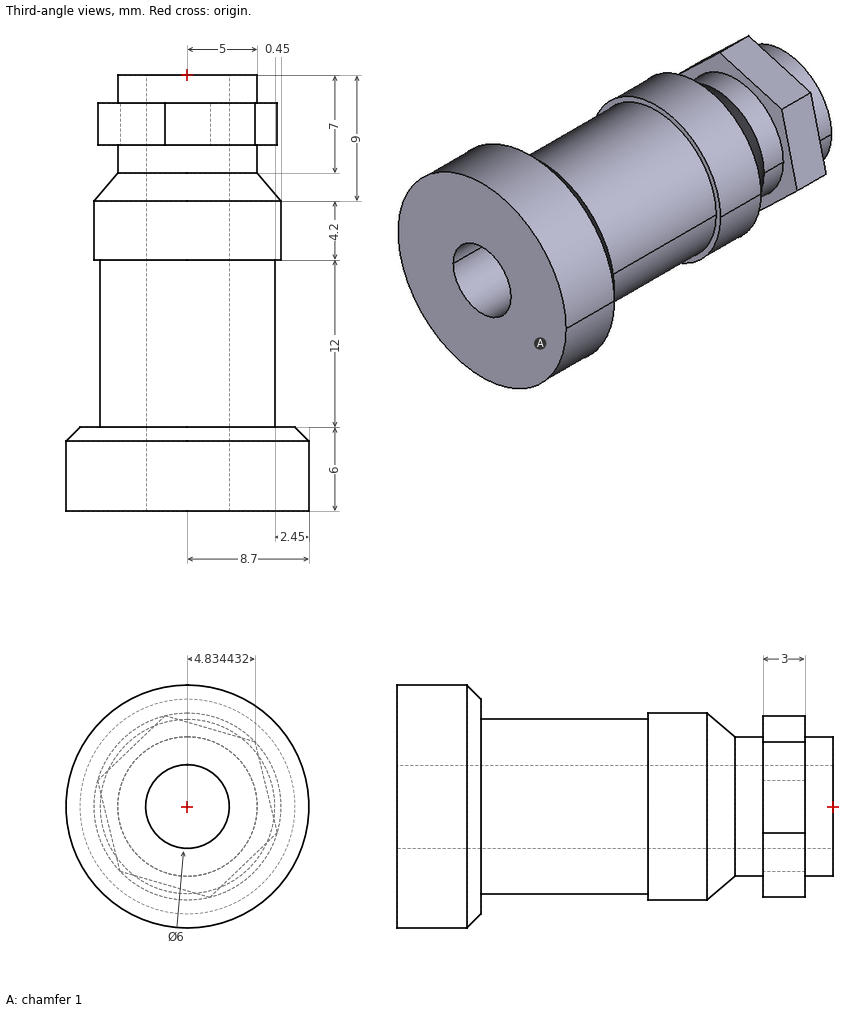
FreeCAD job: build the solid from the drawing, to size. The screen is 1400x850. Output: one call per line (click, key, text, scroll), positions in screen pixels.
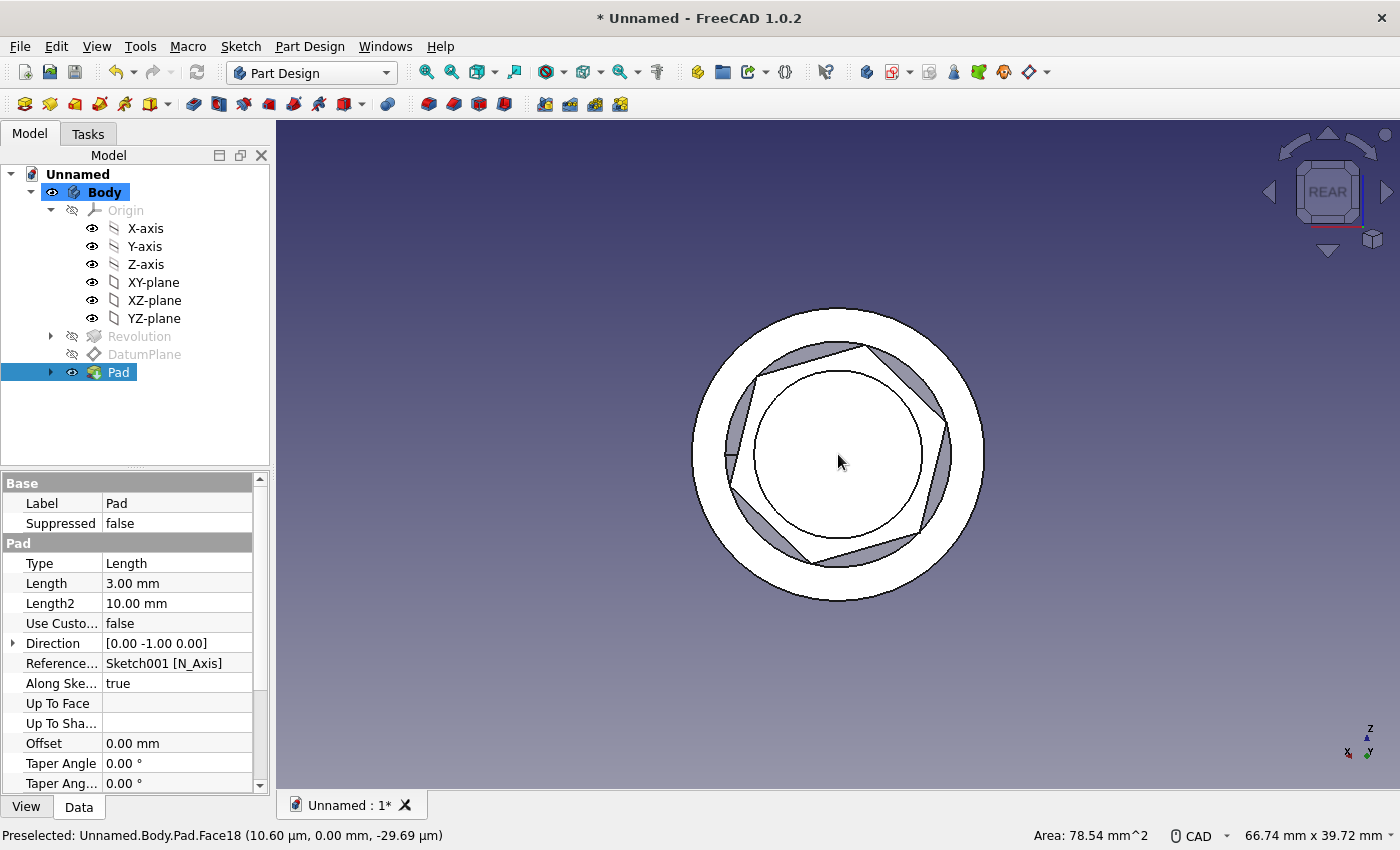
click(892, 72)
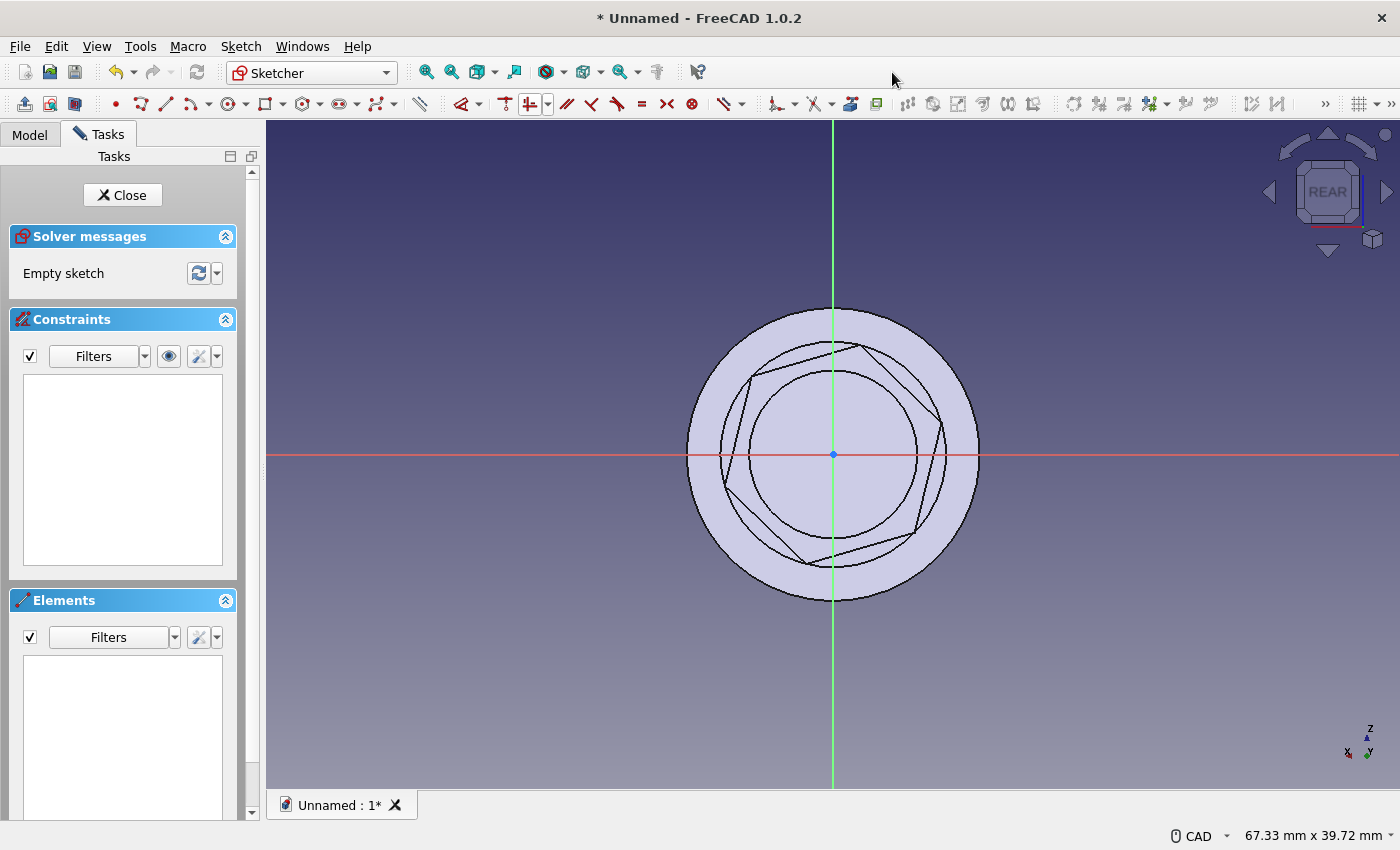
scroll(856, 454, up, 7)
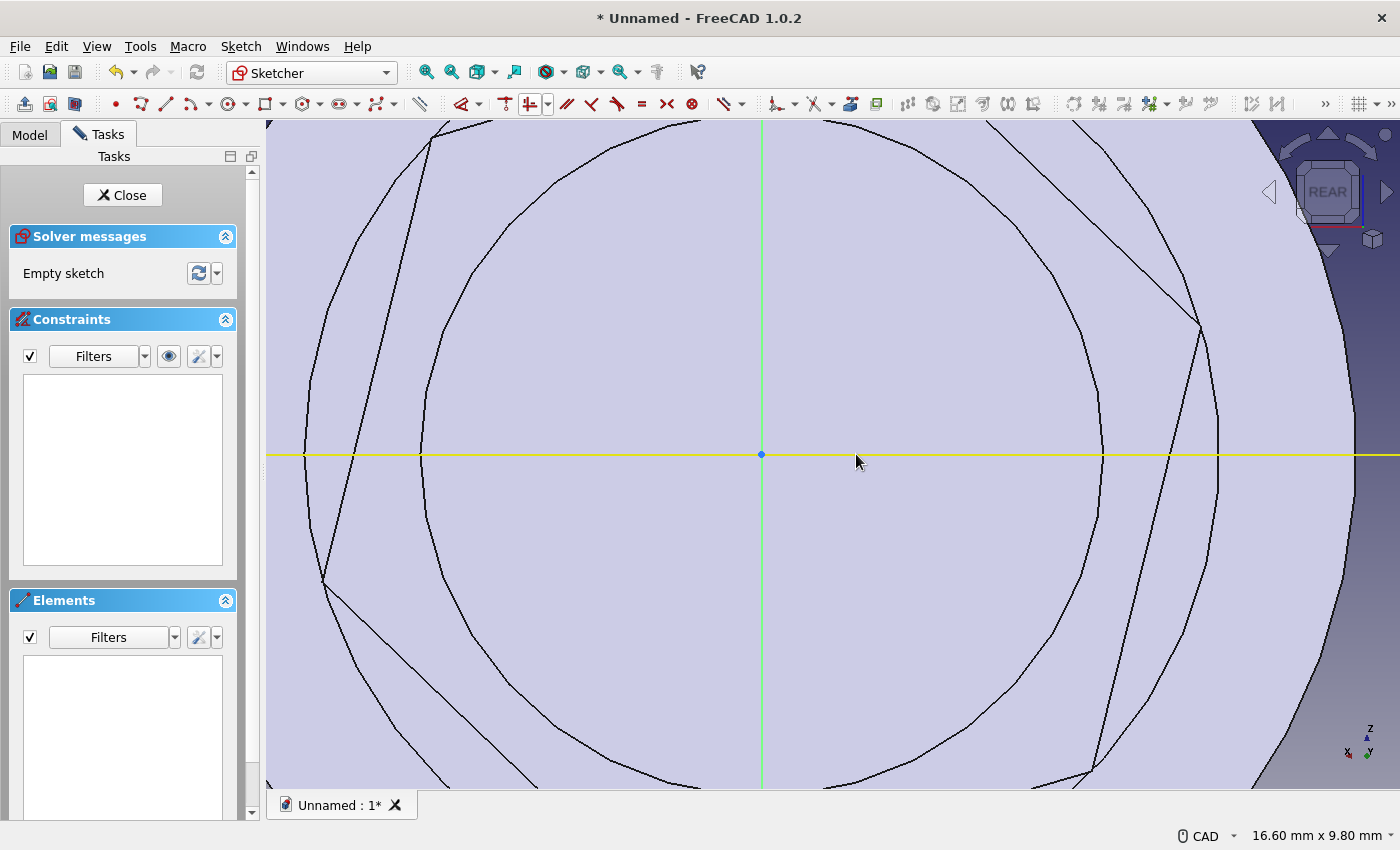
key(g)
key(c)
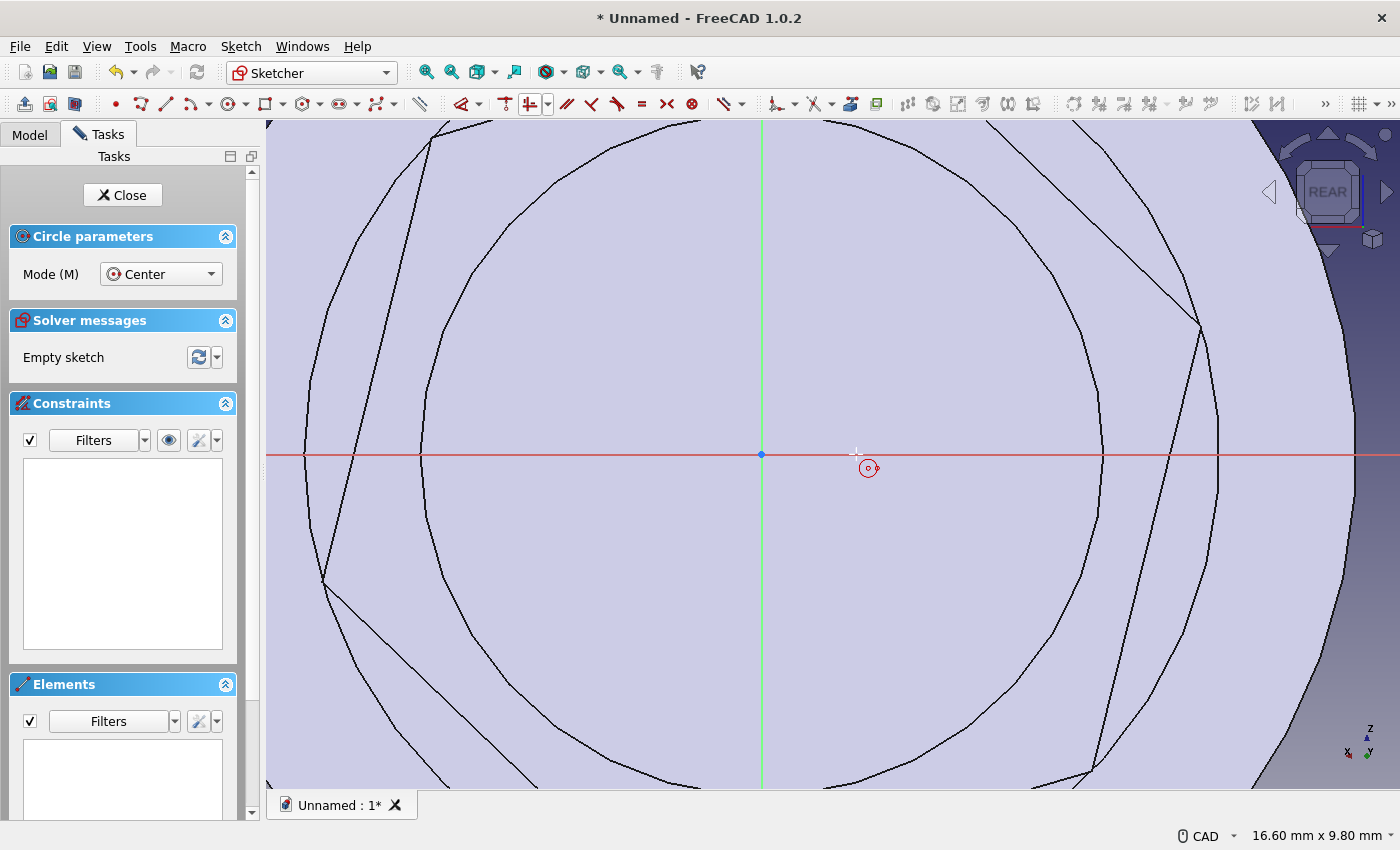
click(762, 454)
click(907, 310)
key(Escape)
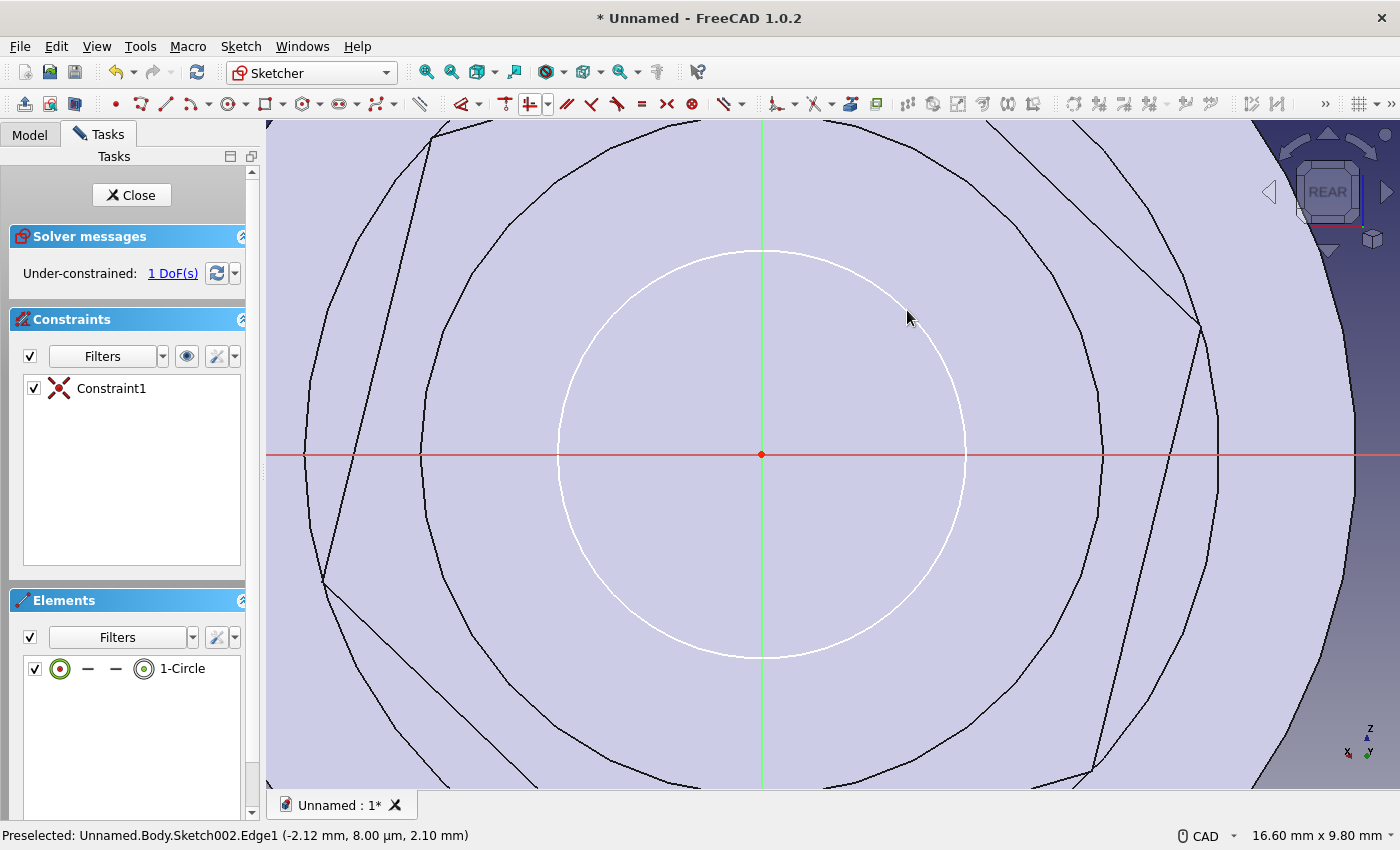
key(d)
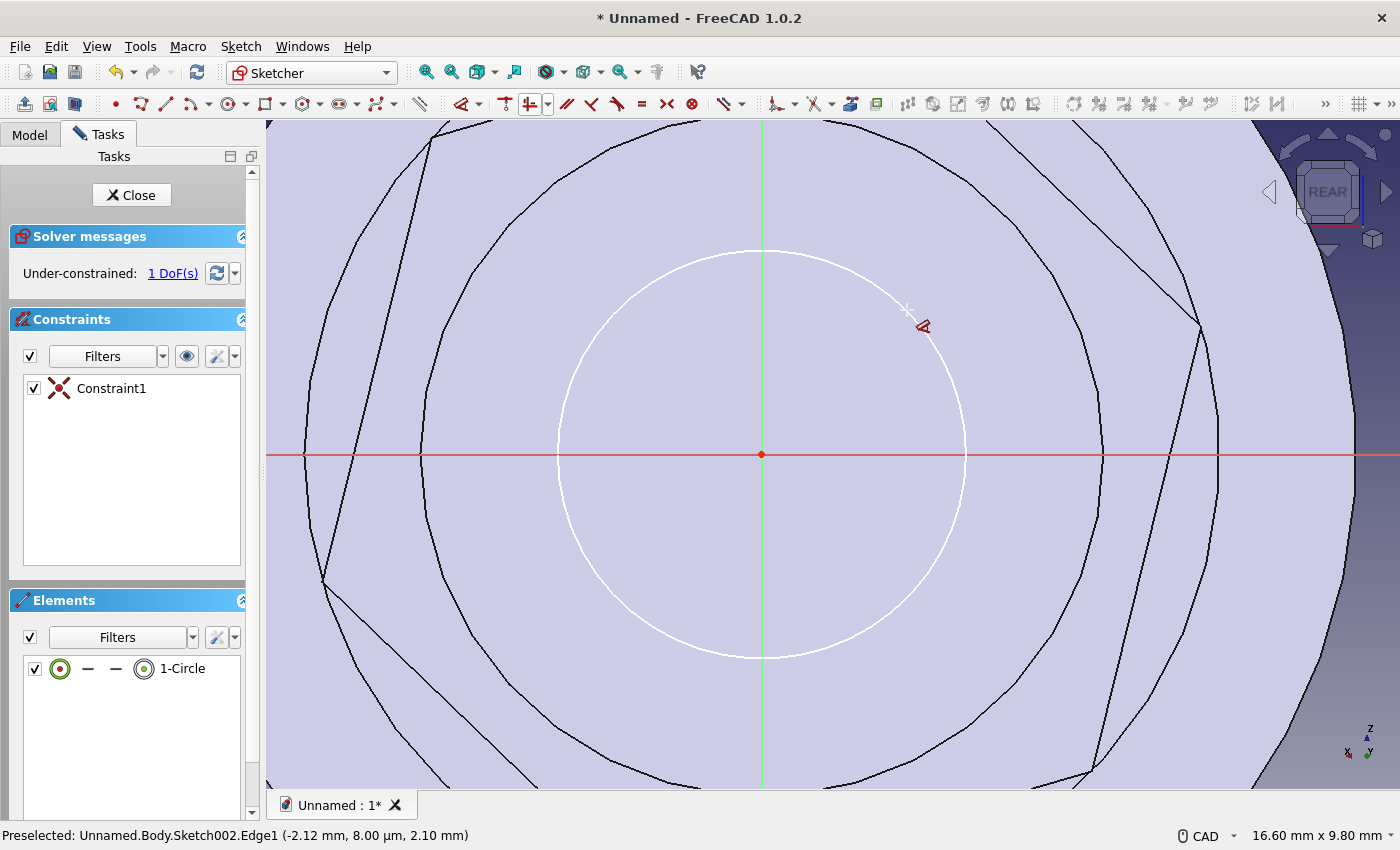
click(906, 310)
click(929, 287)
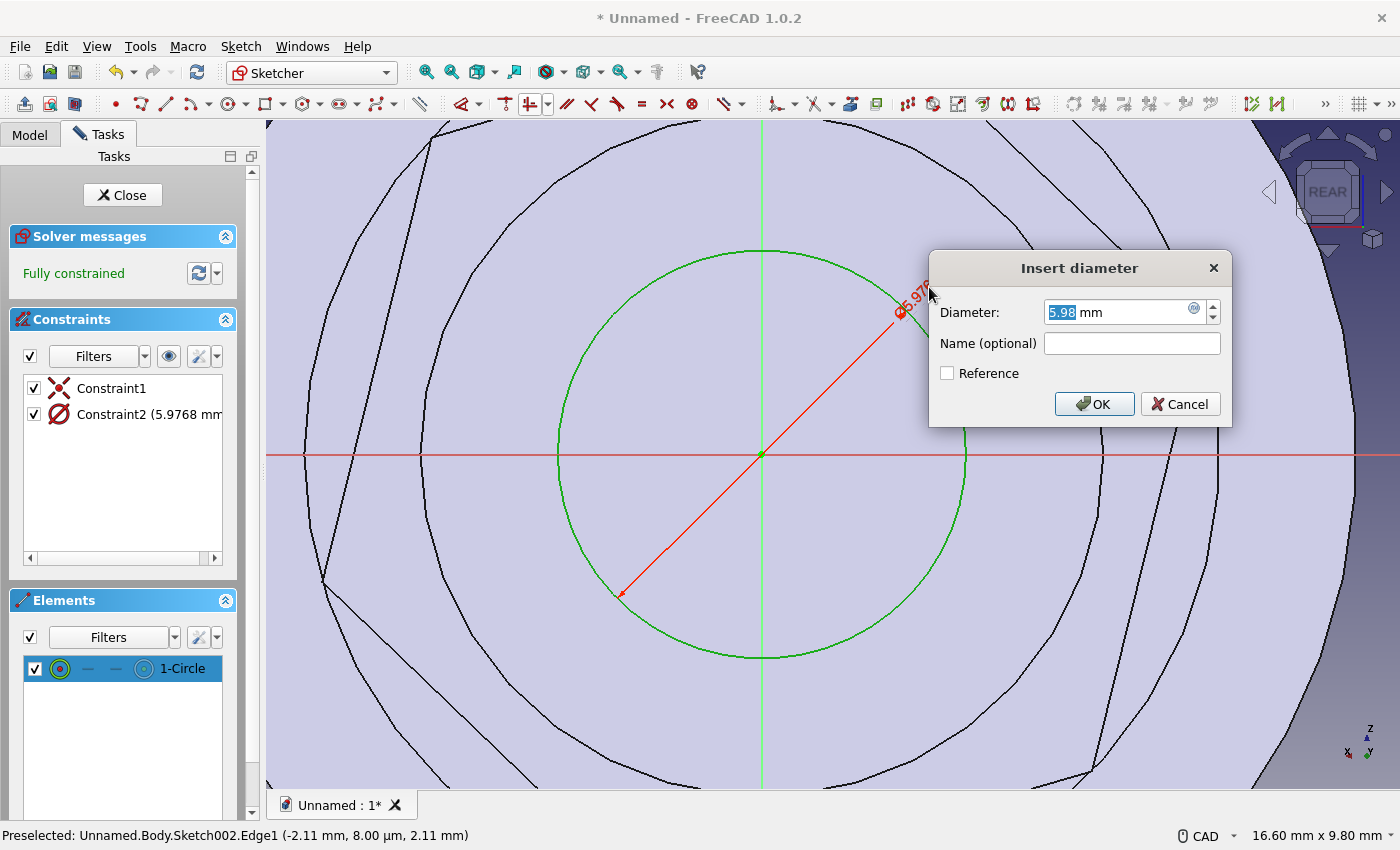
text(6)
key(Return)
key(Escape)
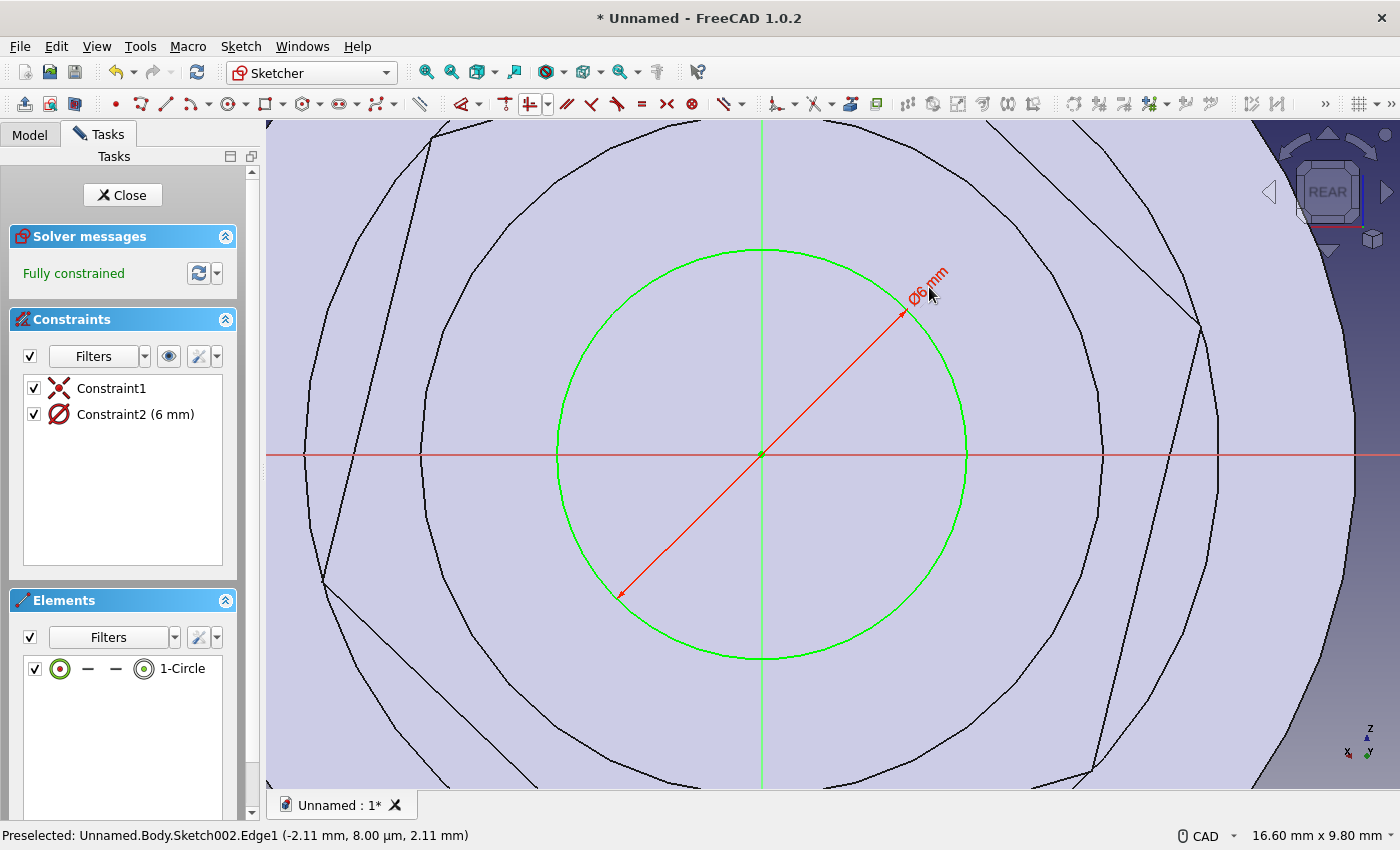
click(123, 195)